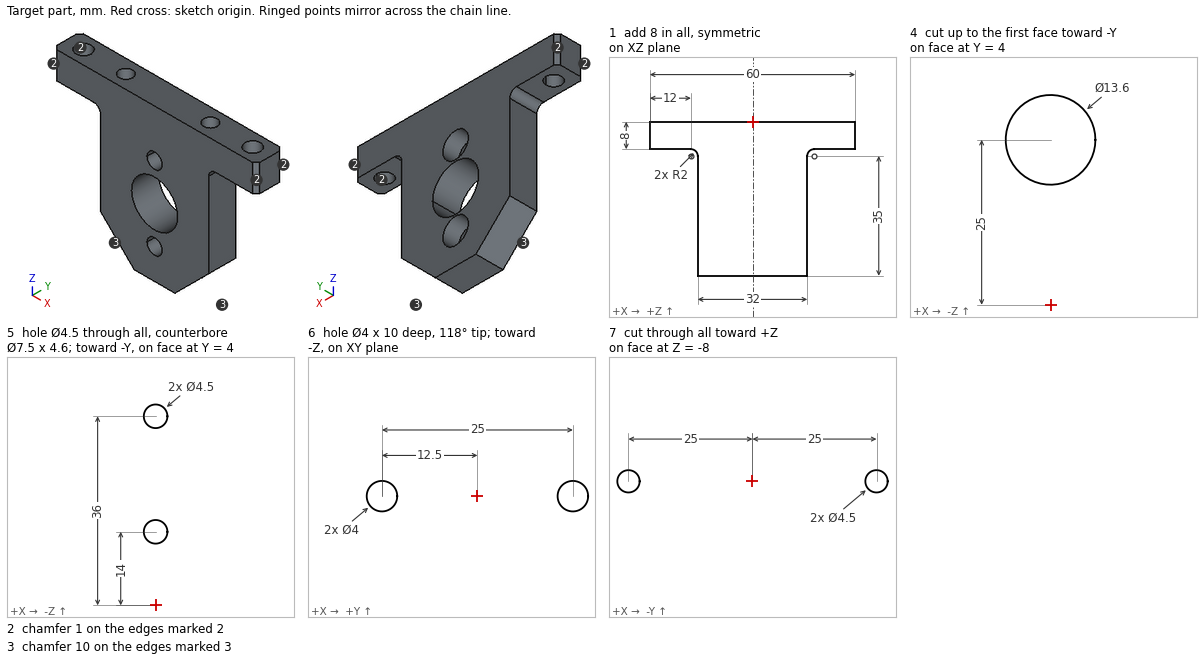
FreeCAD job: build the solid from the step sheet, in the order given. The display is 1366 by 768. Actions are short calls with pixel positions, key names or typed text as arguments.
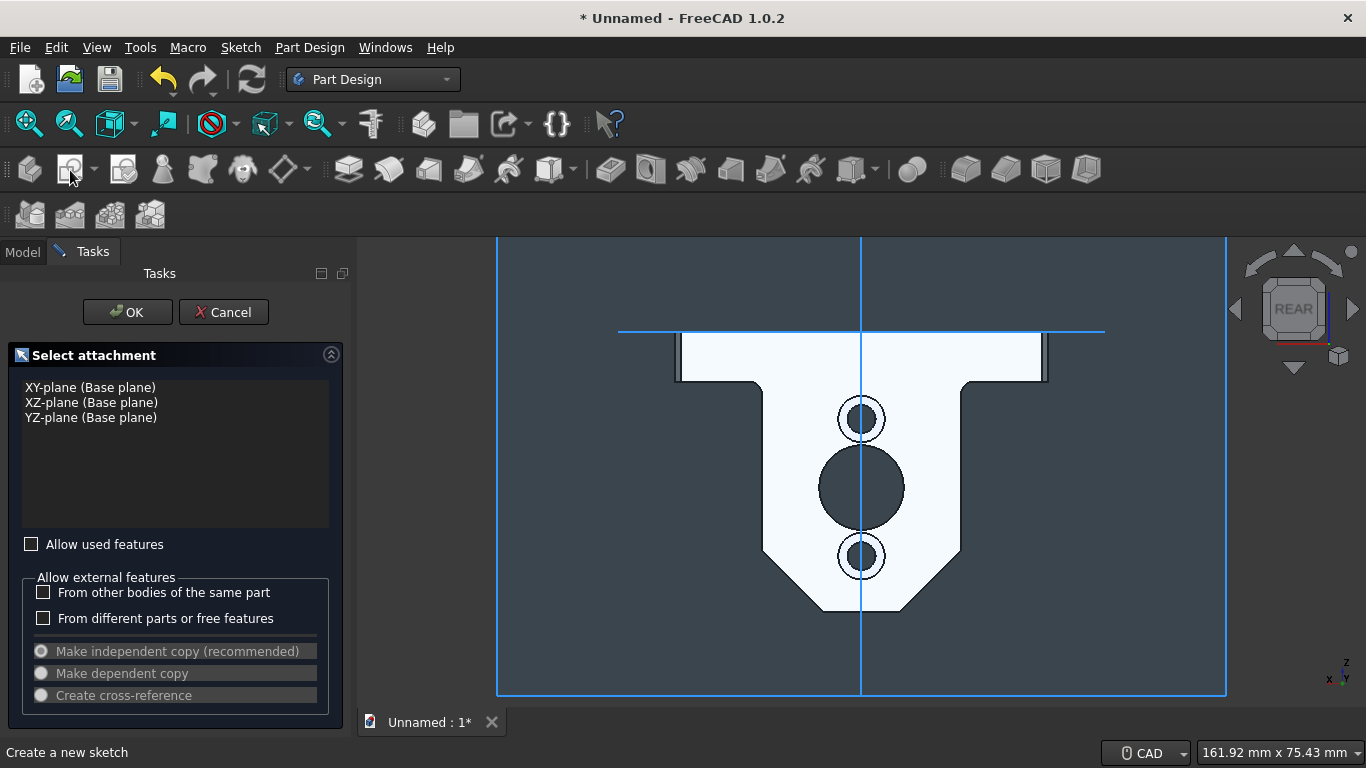
click(82, 388)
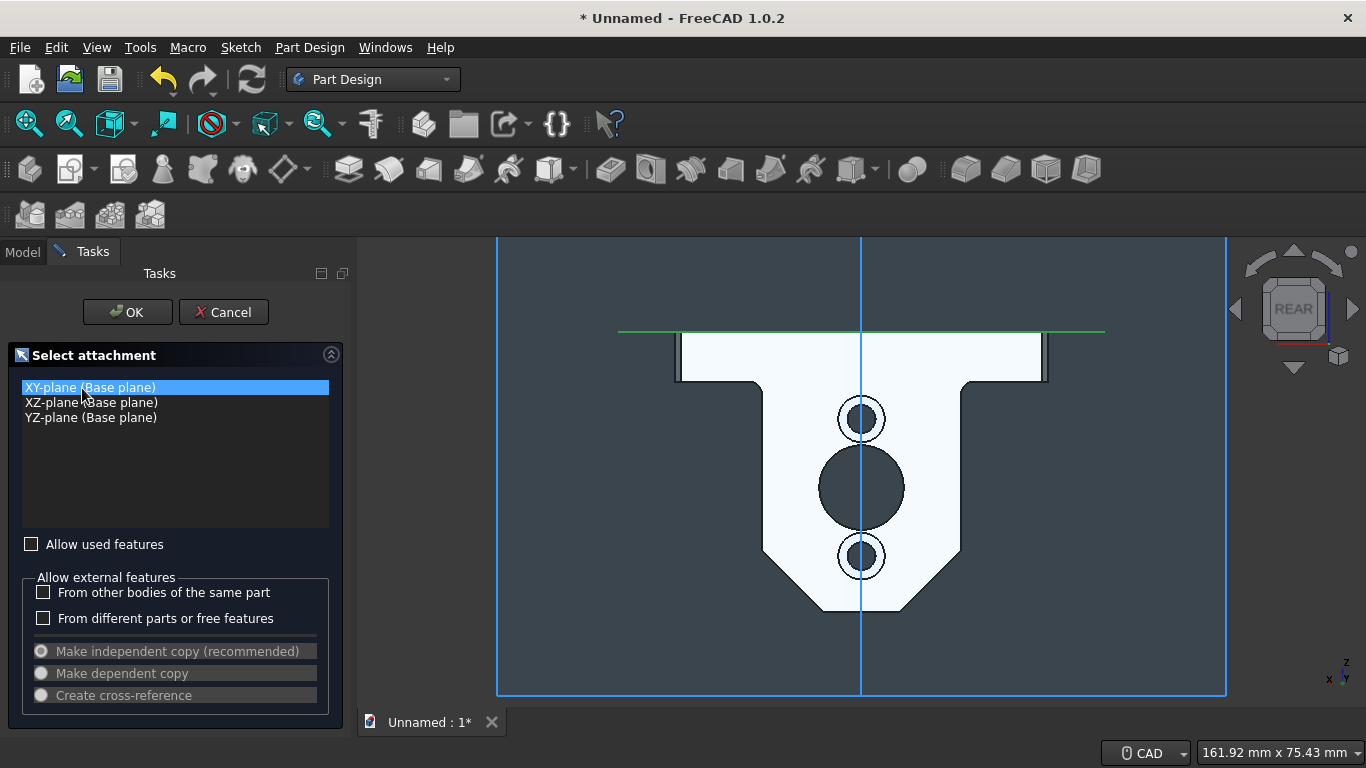
click(128, 312)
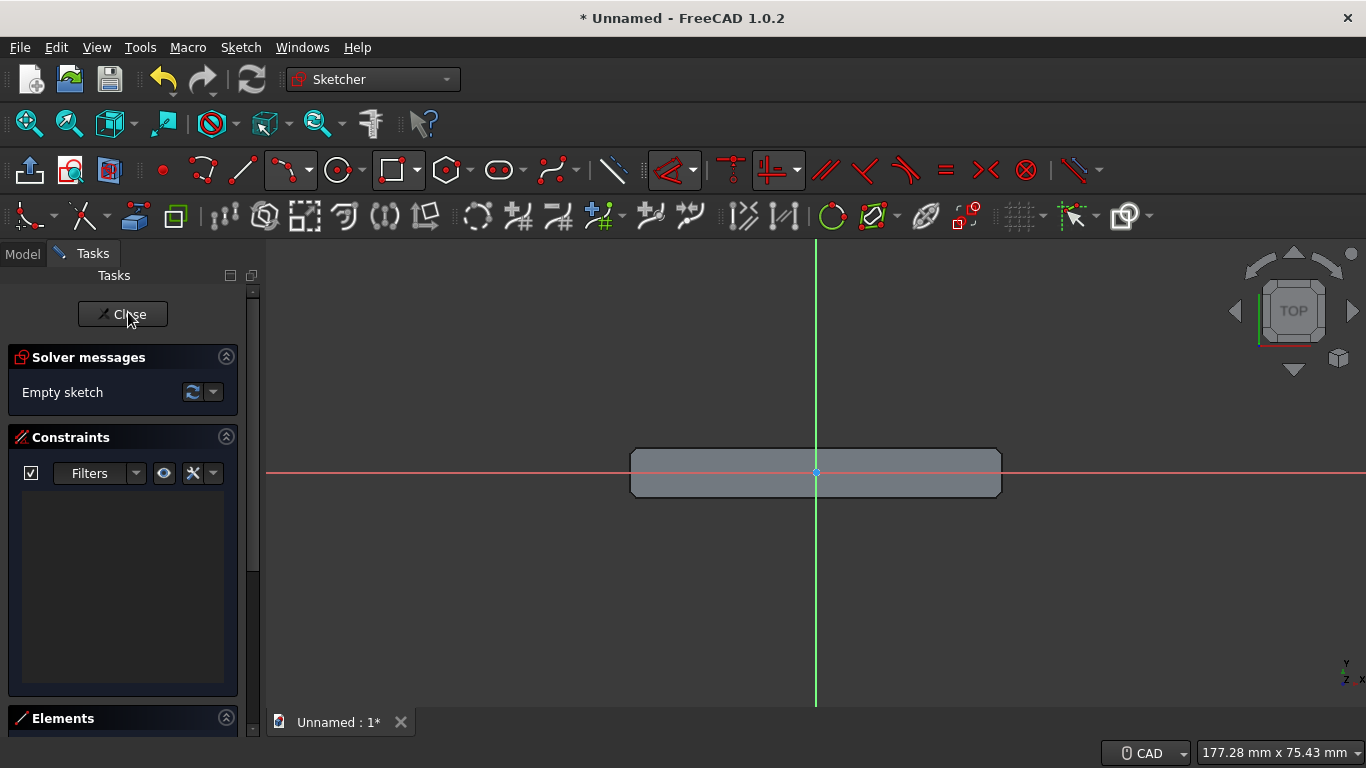
scroll(846, 473, up, 6)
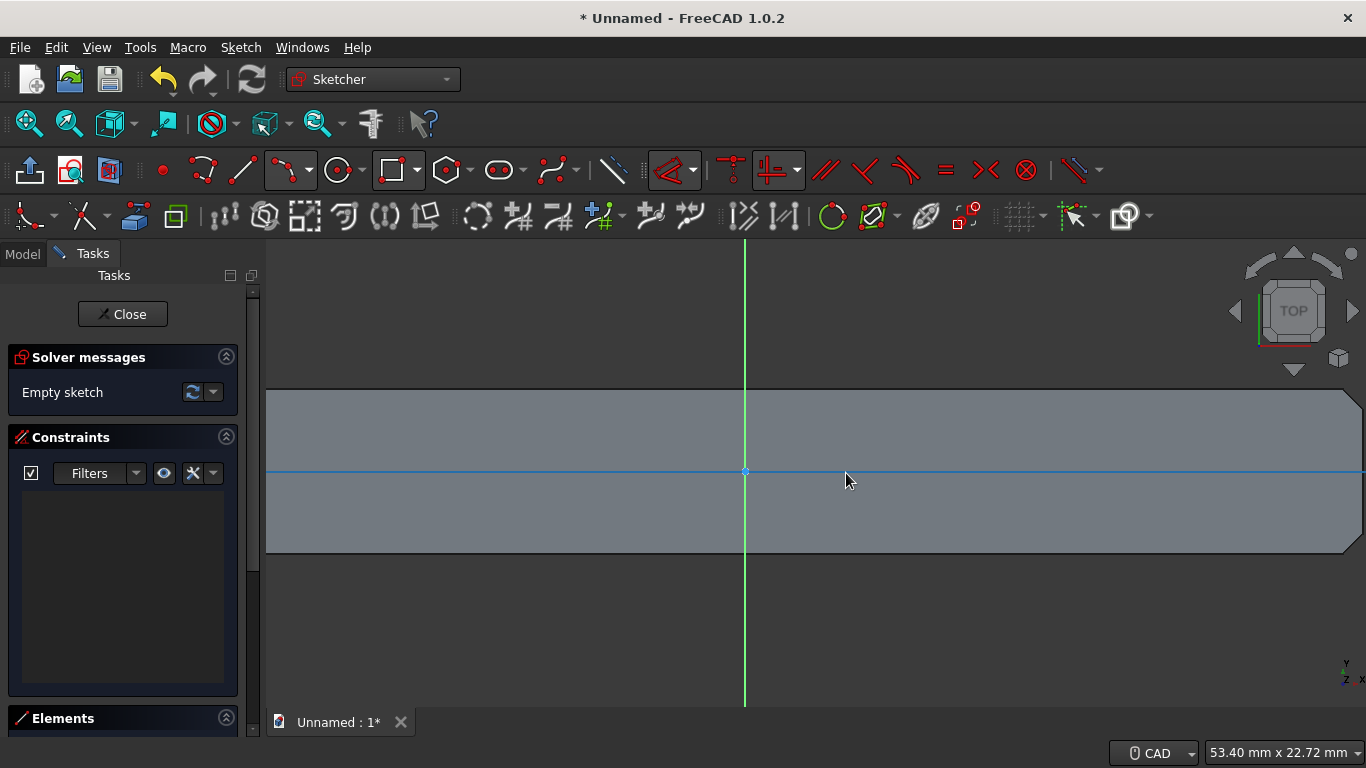
click(338, 170)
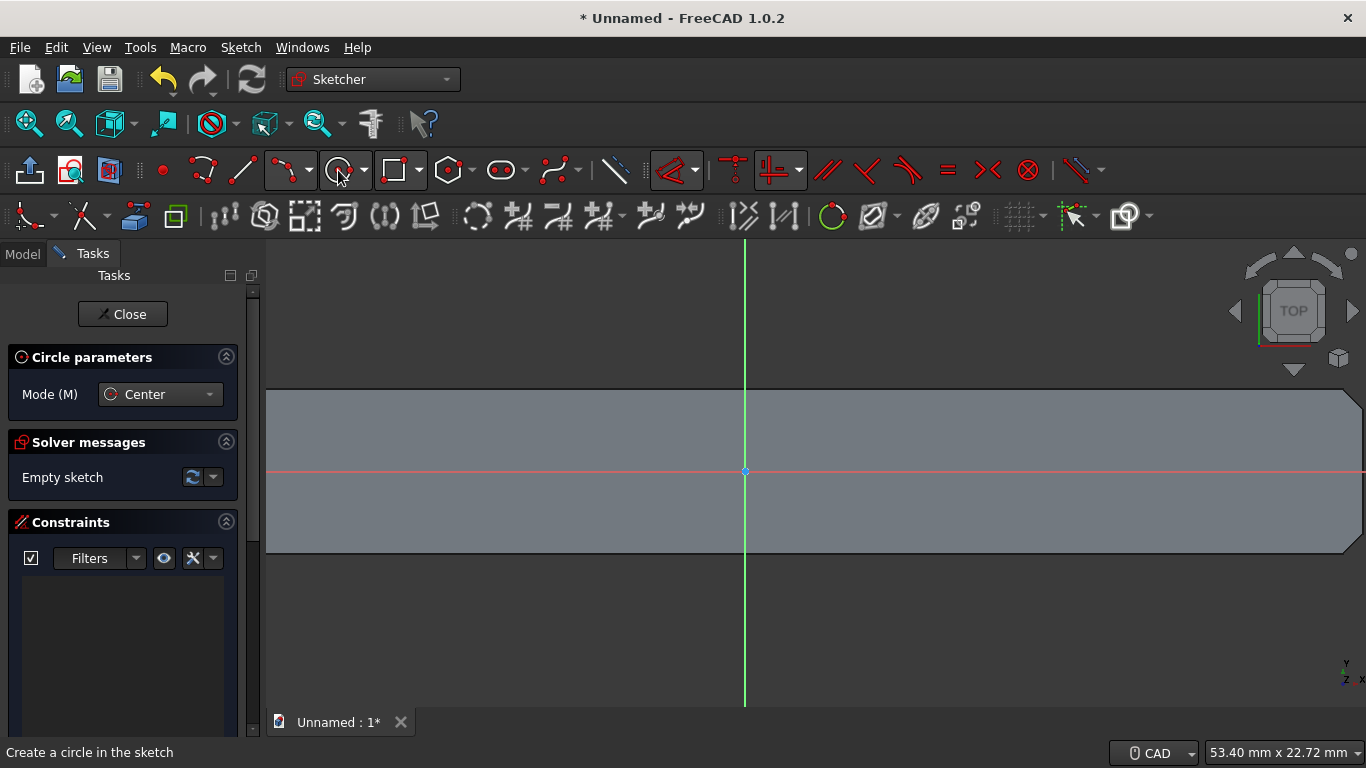
click(488, 472)
click(517, 443)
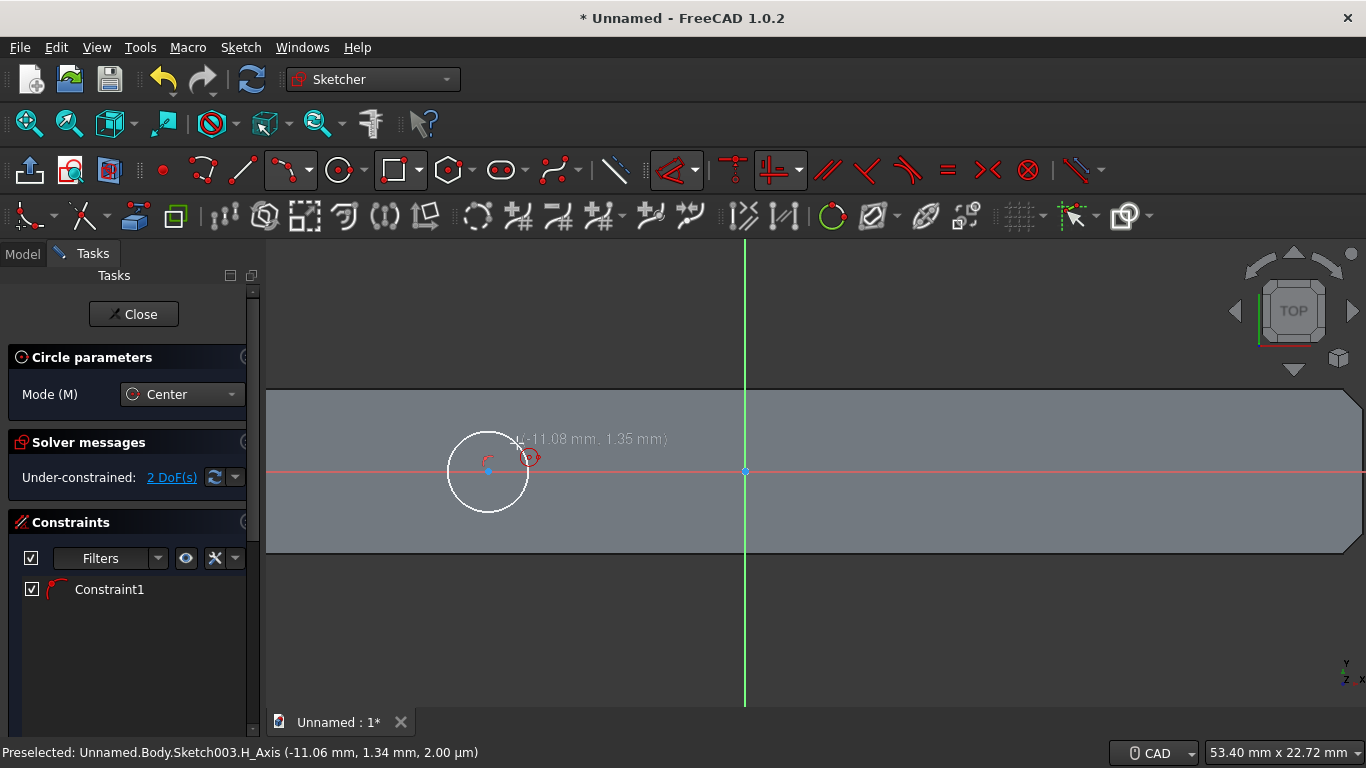
click(1003, 472)
click(1032, 443)
key(Escape)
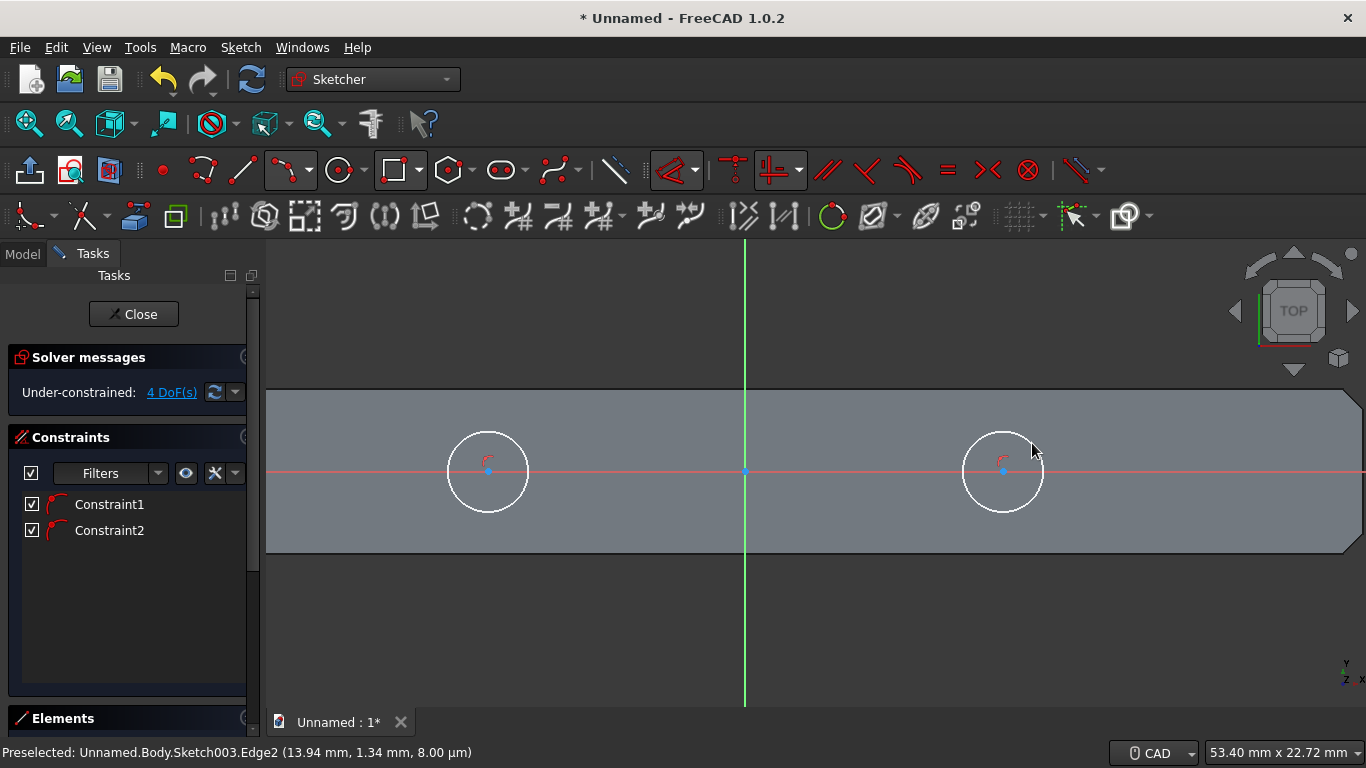
click(516, 443)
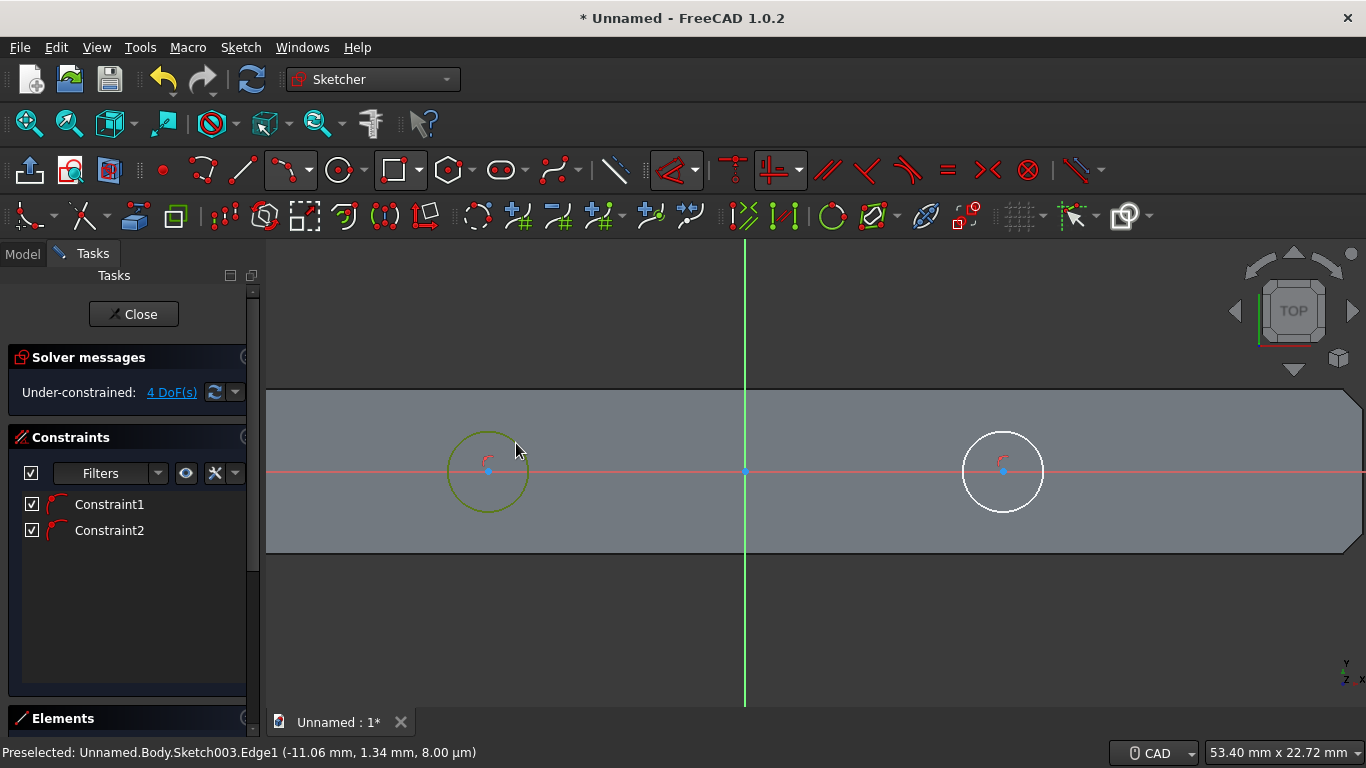
click(1031, 443)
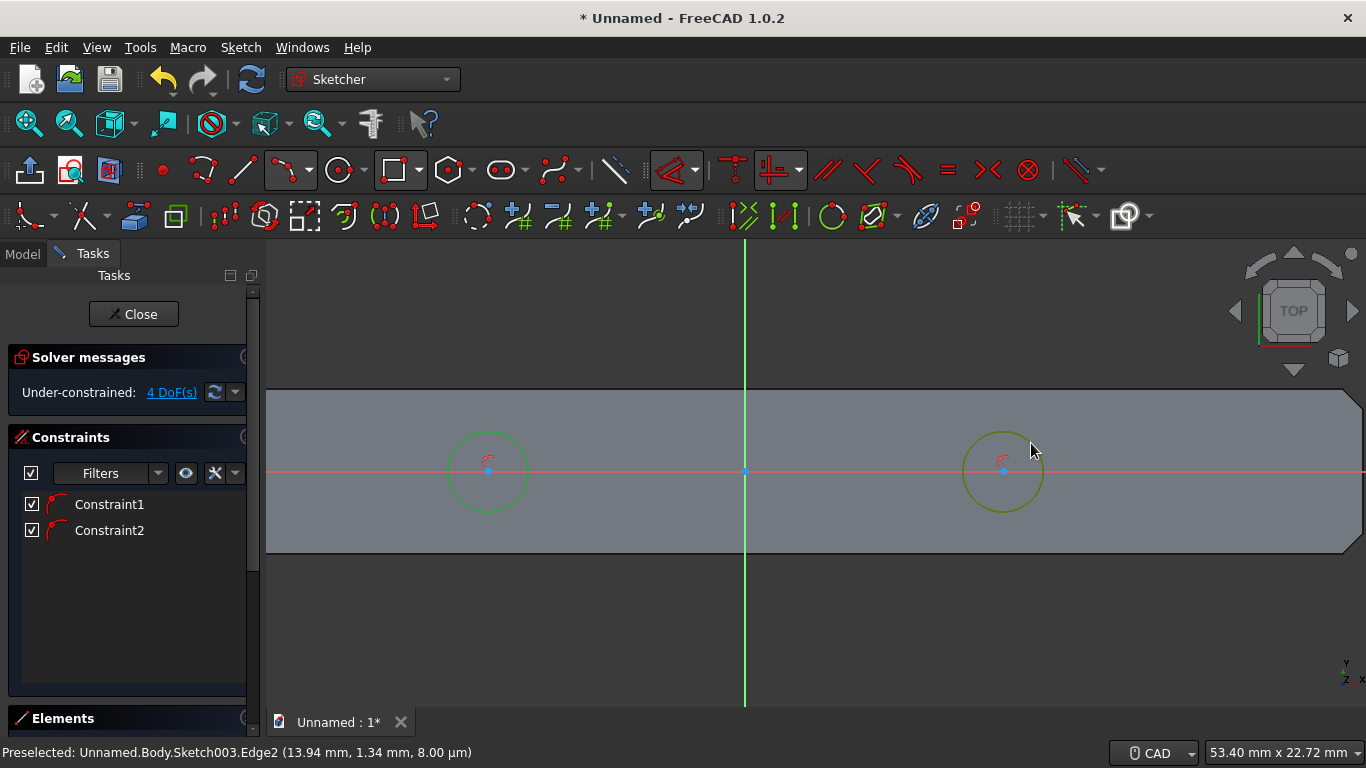
click(948, 170)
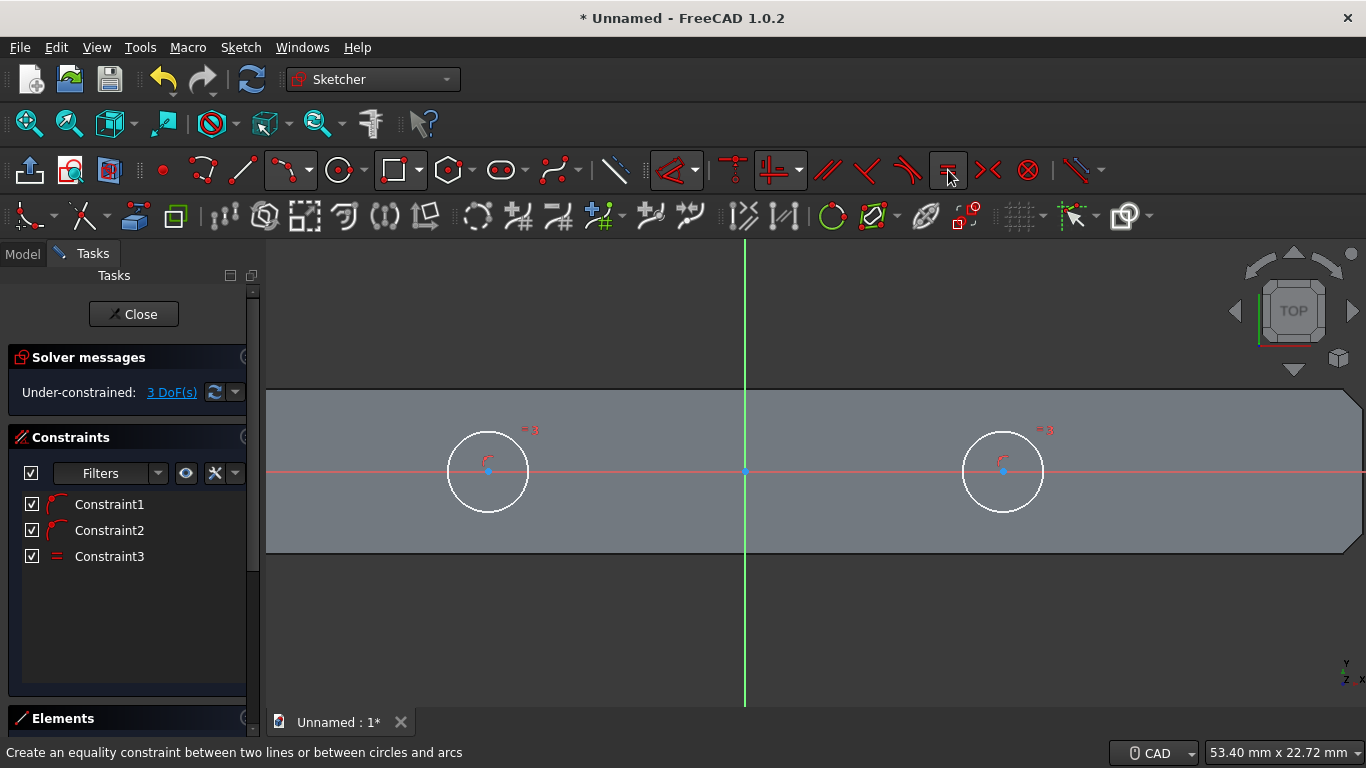
click(516, 443)